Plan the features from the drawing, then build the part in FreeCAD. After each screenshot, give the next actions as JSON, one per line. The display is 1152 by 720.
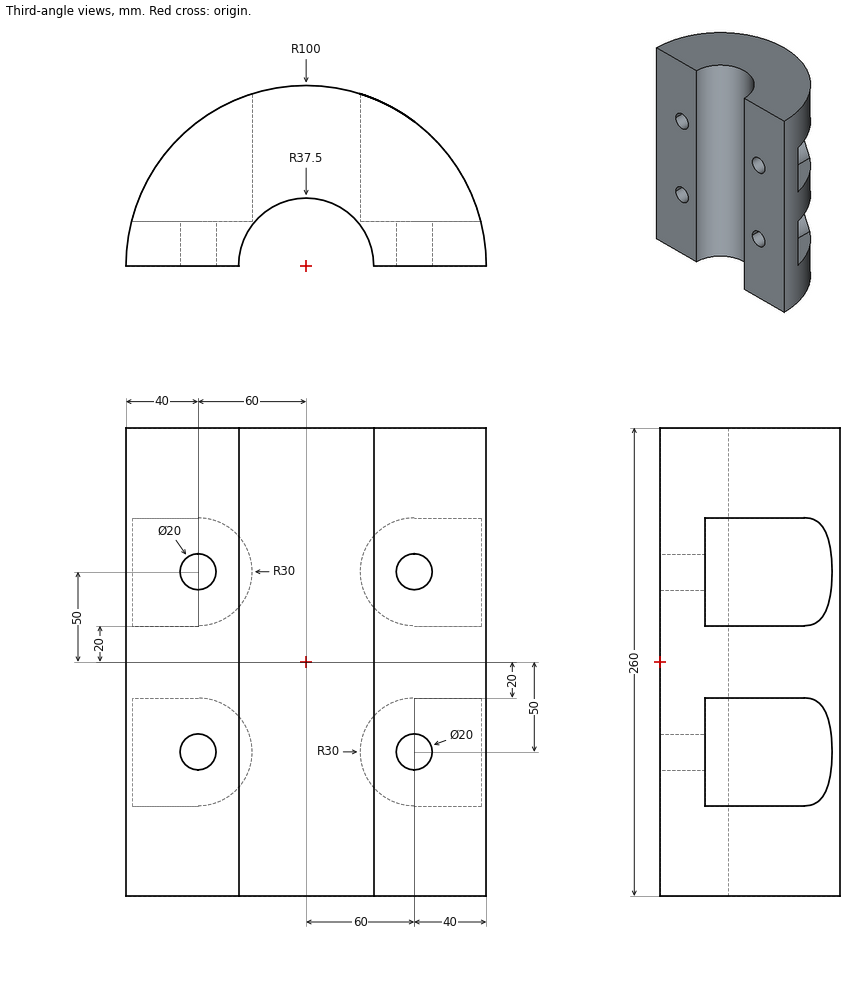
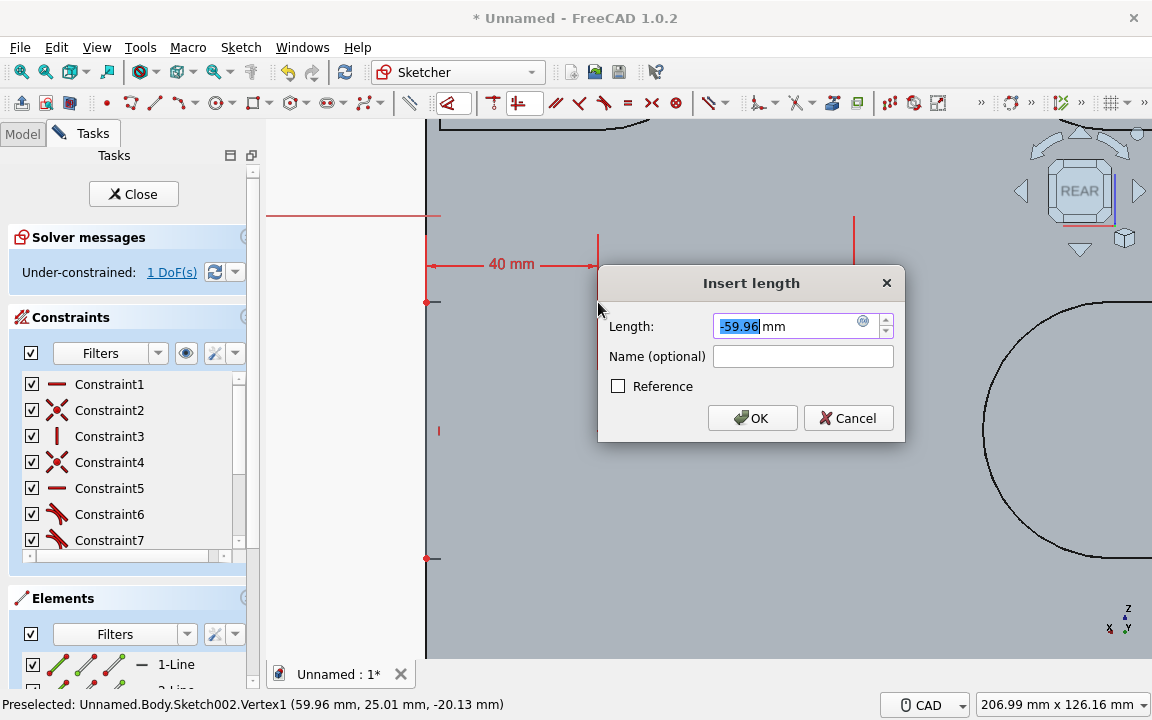
{"action": "type", "text": "-60"}
{"action": "key", "text": "Return"}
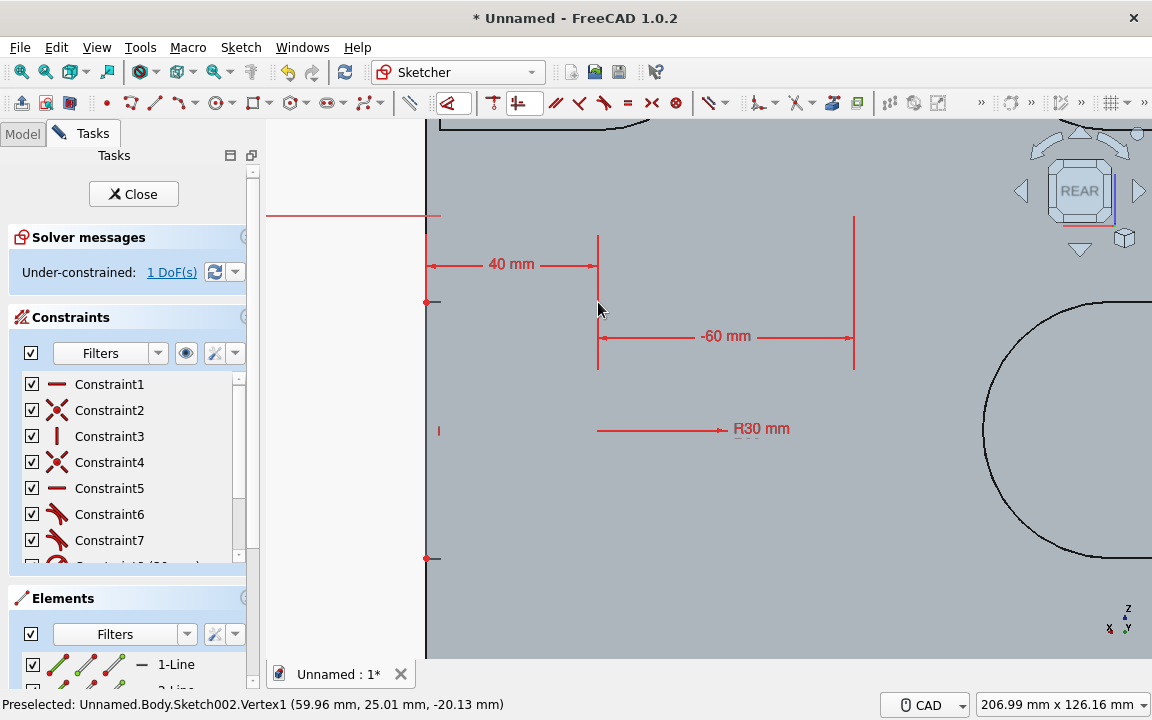
{"action": "left_click", "coordinate": [598, 302]}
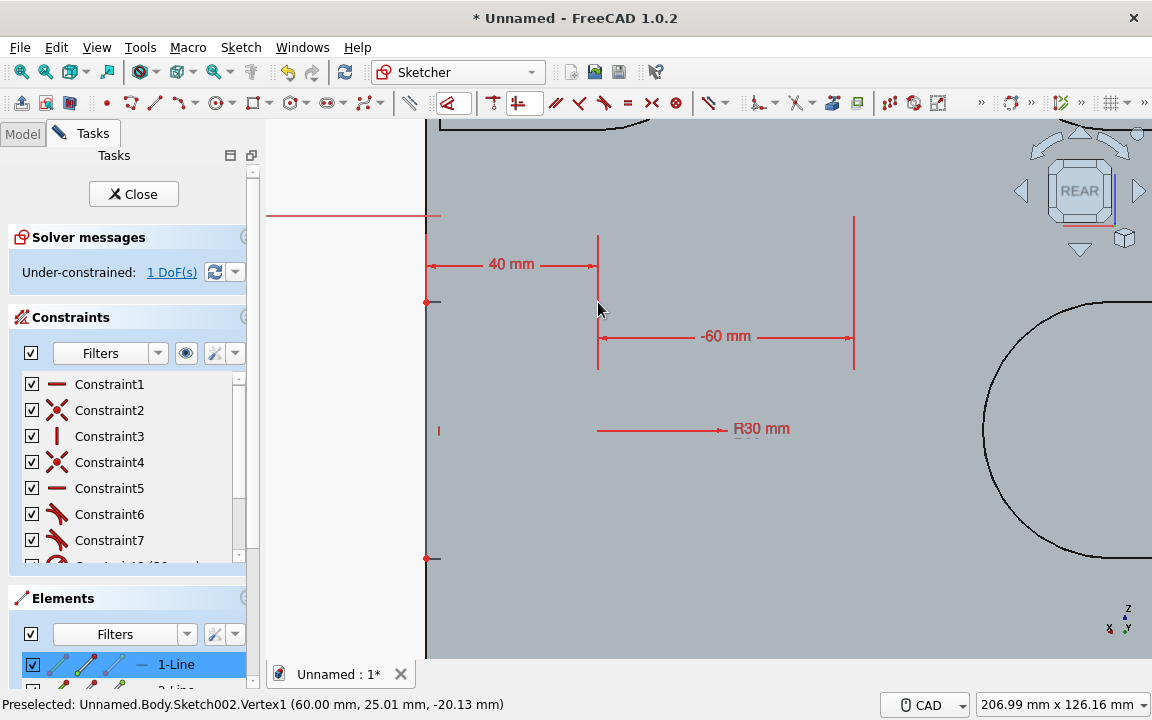
{"action": "key", "text": "i"}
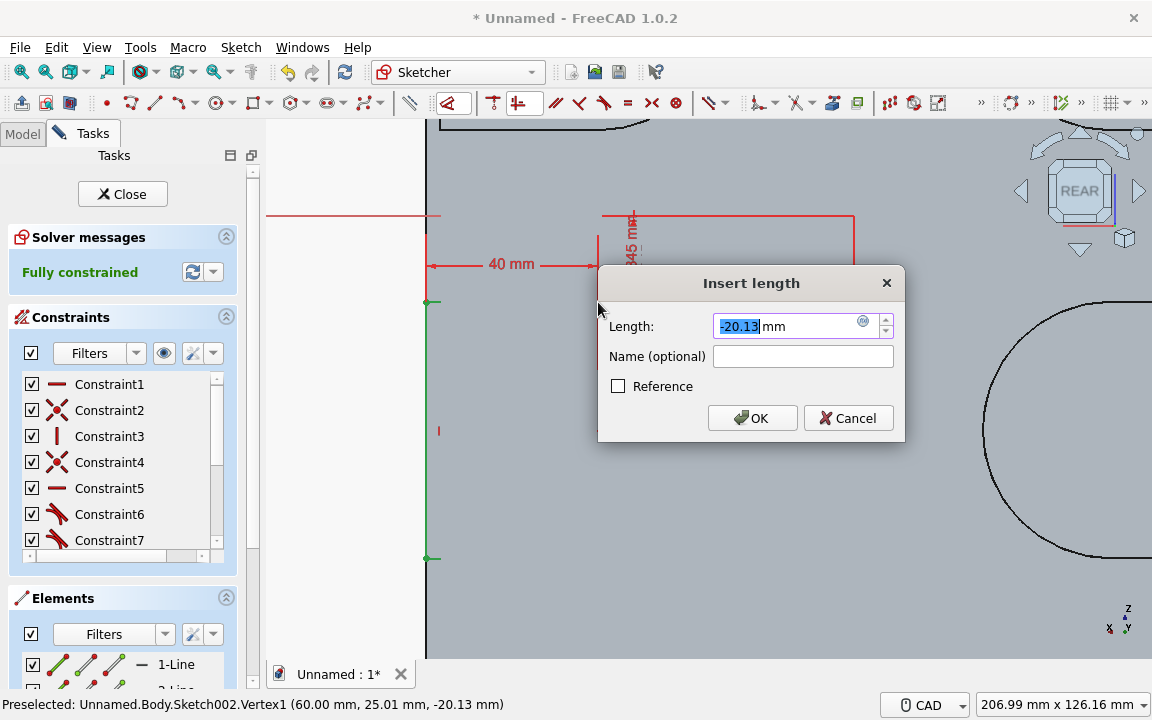
{"action": "type", "text": "-20"}
{"action": "key", "text": "Return"}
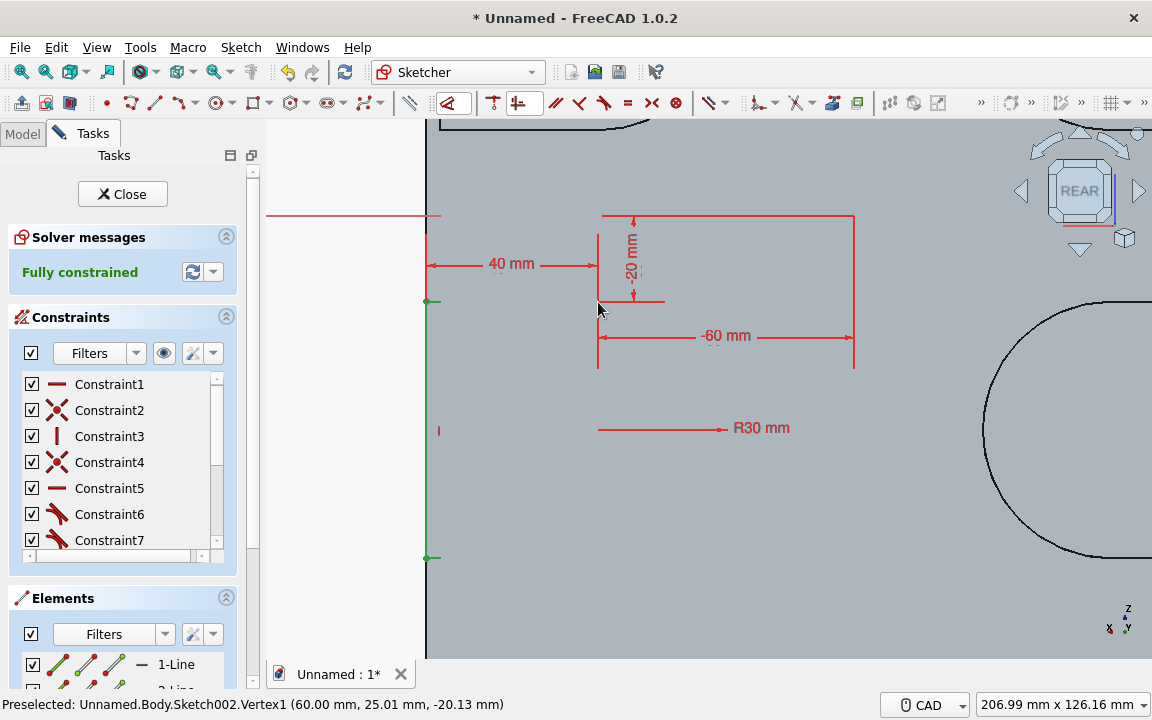
{"action": "left_click", "coordinate": [123, 194]}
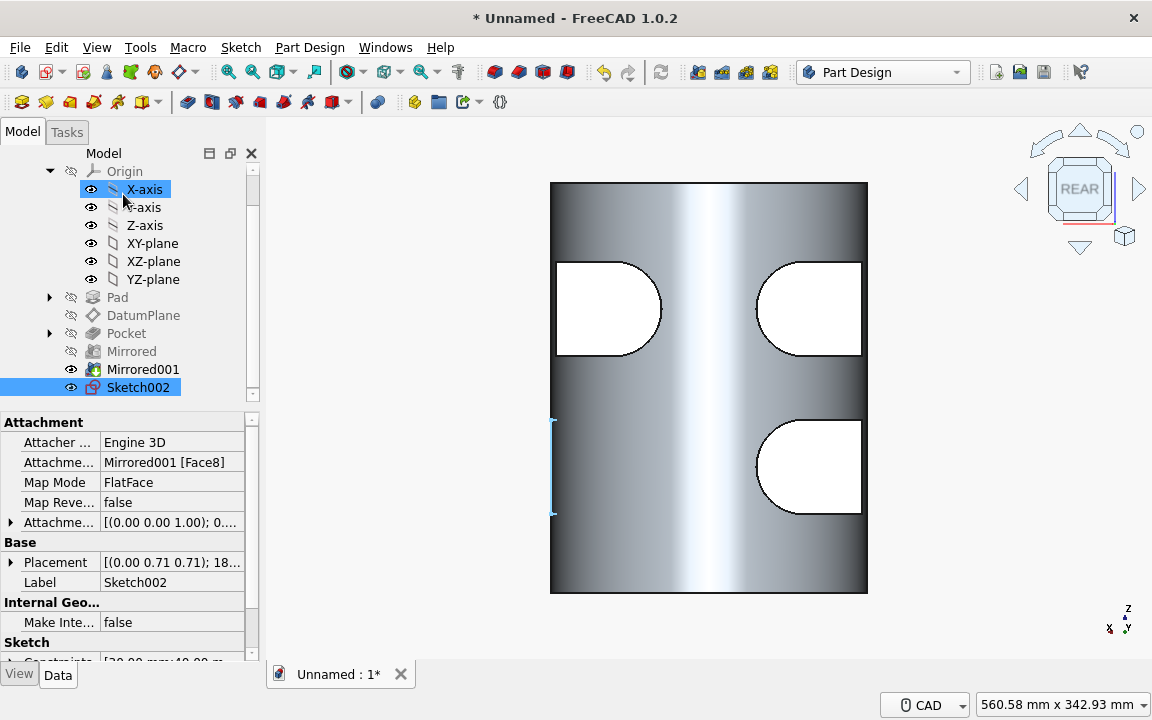
{"action": "left_click", "coordinate": [188, 102]}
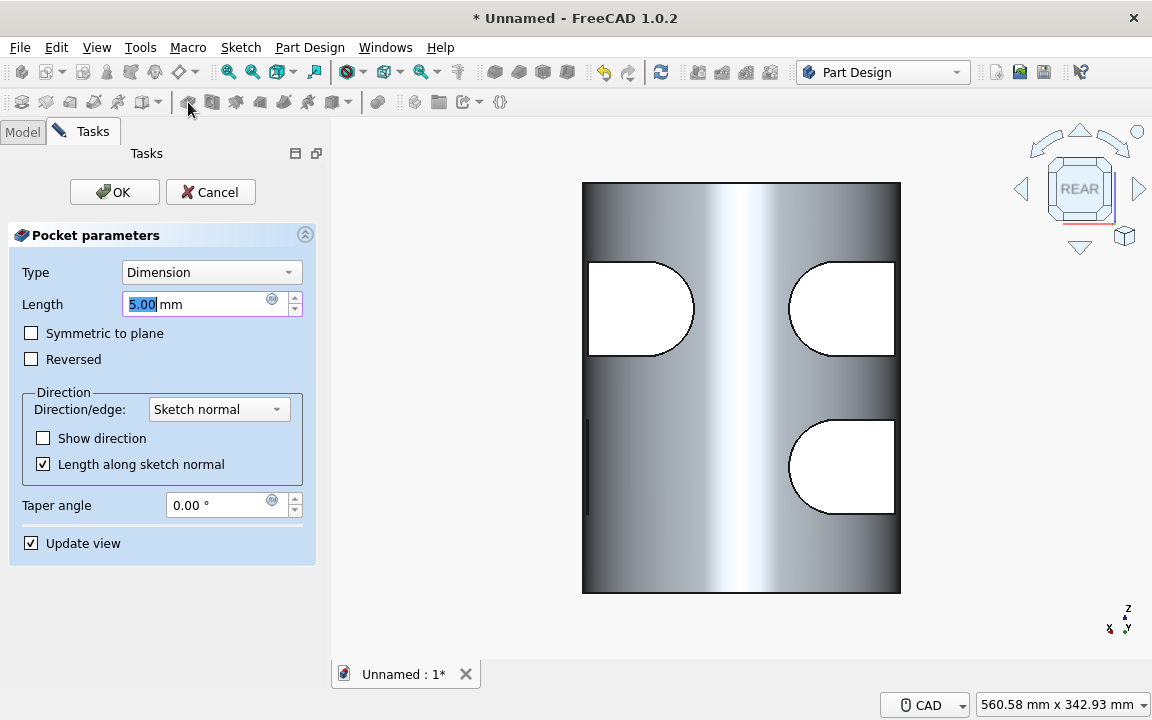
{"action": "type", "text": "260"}
{"action": "key", "text": "Tab"}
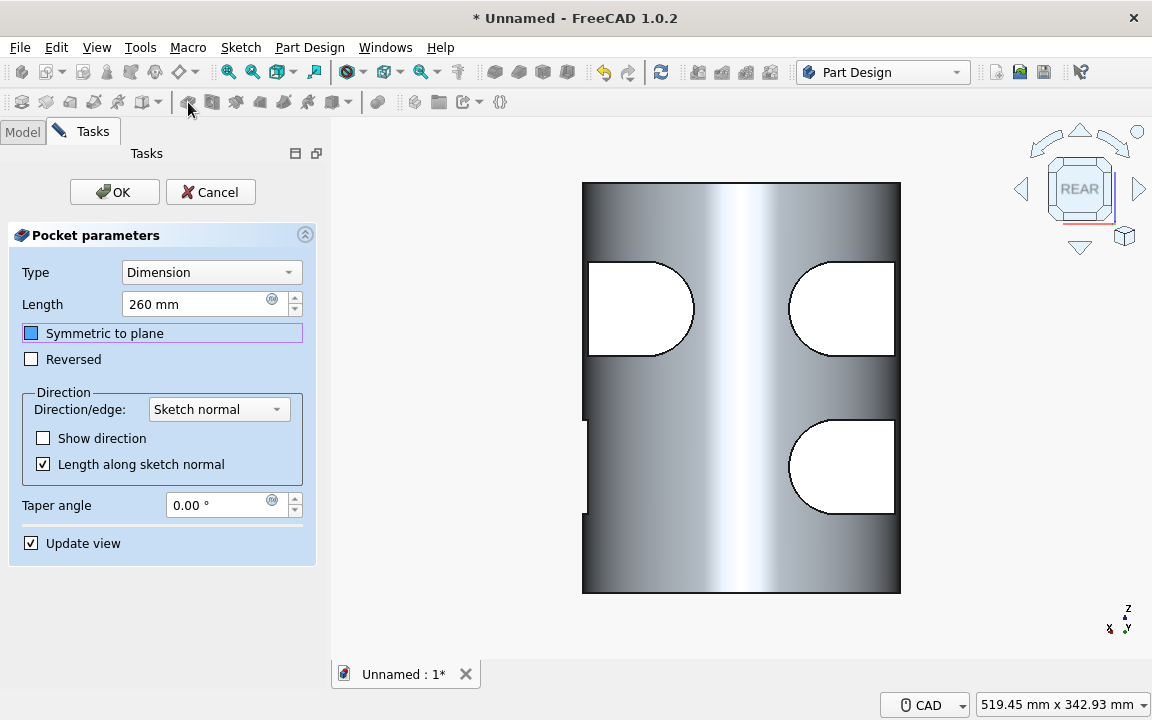
{"action": "left_click", "coordinate": [30, 359]}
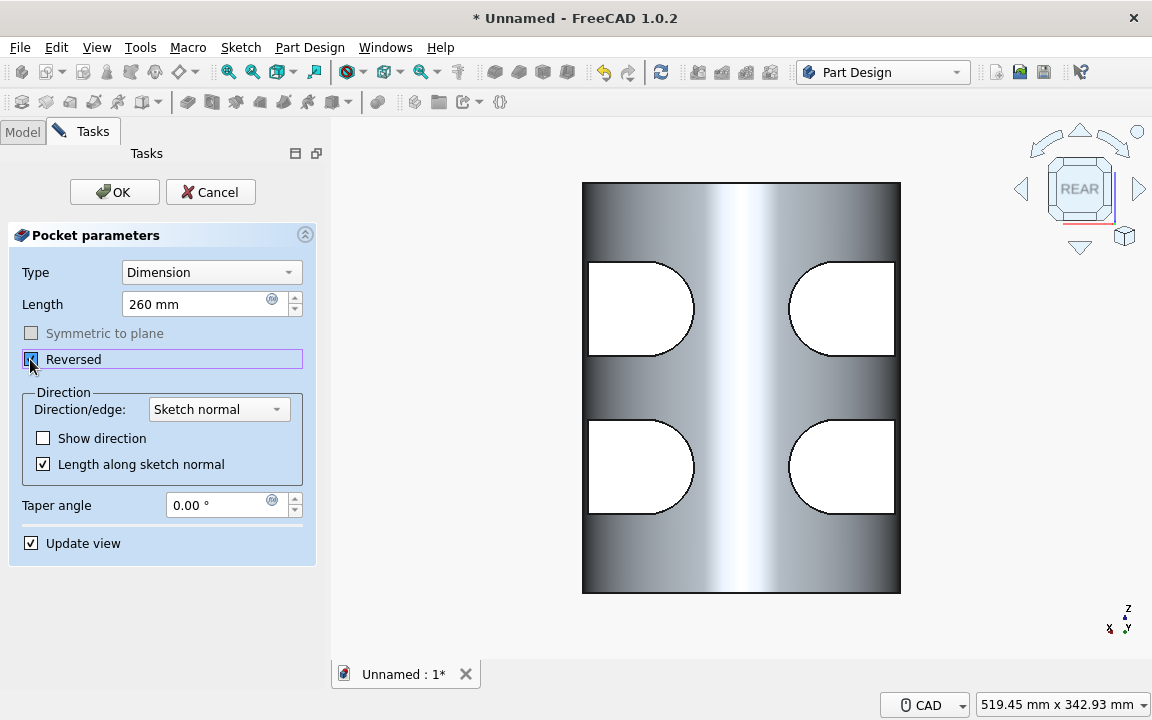
{"action": "left_click", "coordinate": [115, 192]}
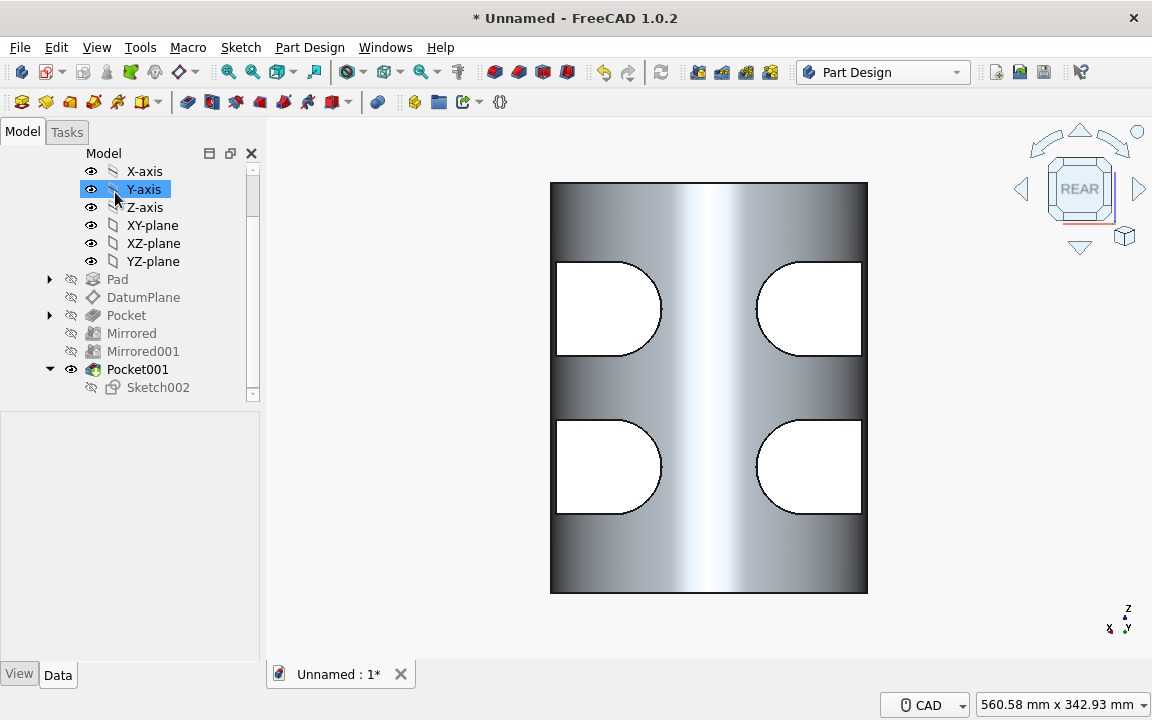
{"action": "left_click", "coordinate": [609, 308]}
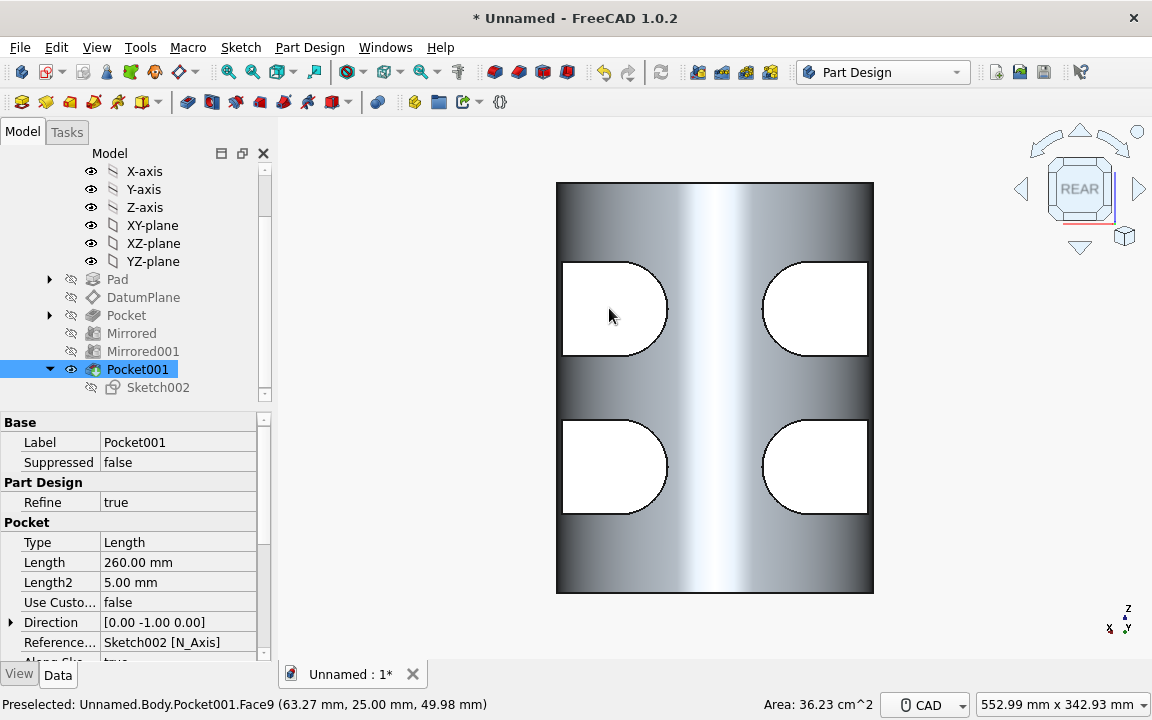
{"action": "left_click", "coordinate": [46, 72]}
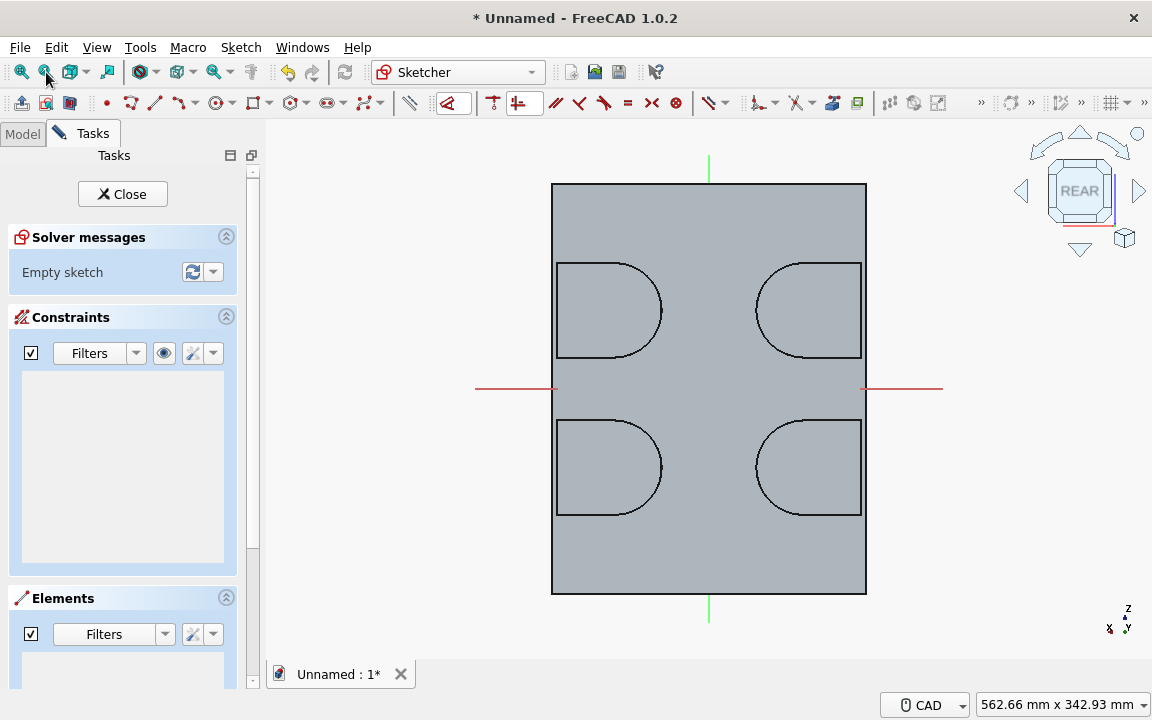
{"action": "key", "text": "q s"}